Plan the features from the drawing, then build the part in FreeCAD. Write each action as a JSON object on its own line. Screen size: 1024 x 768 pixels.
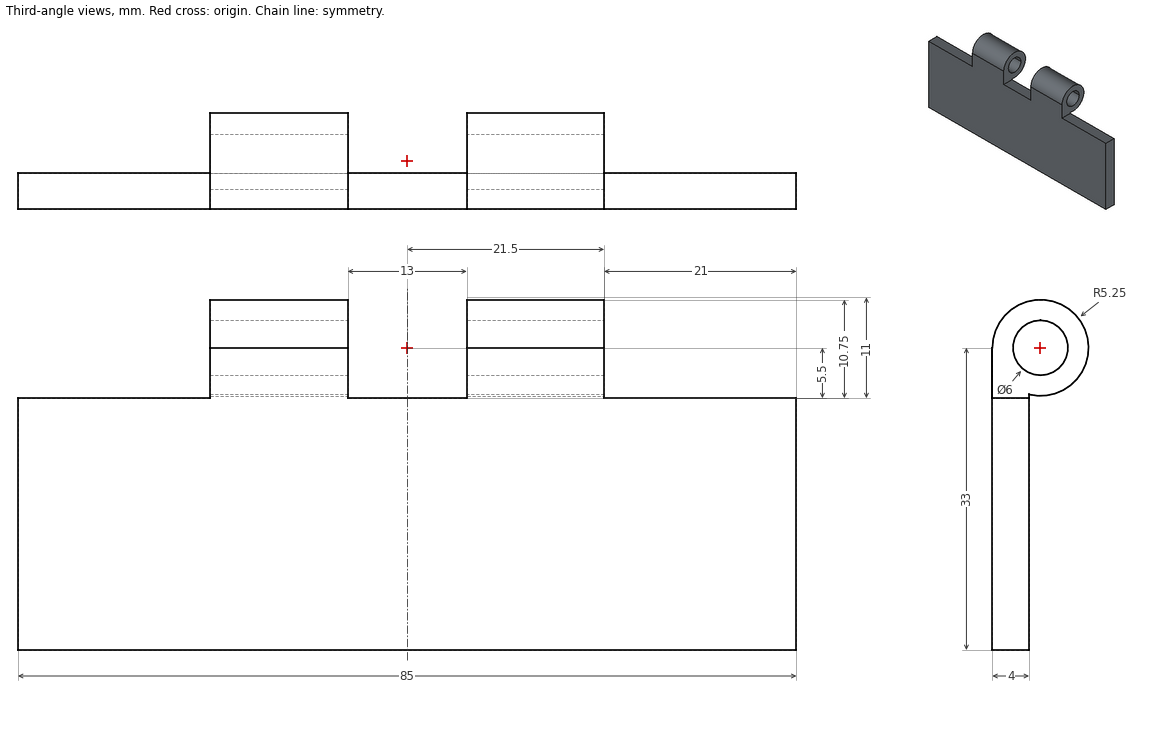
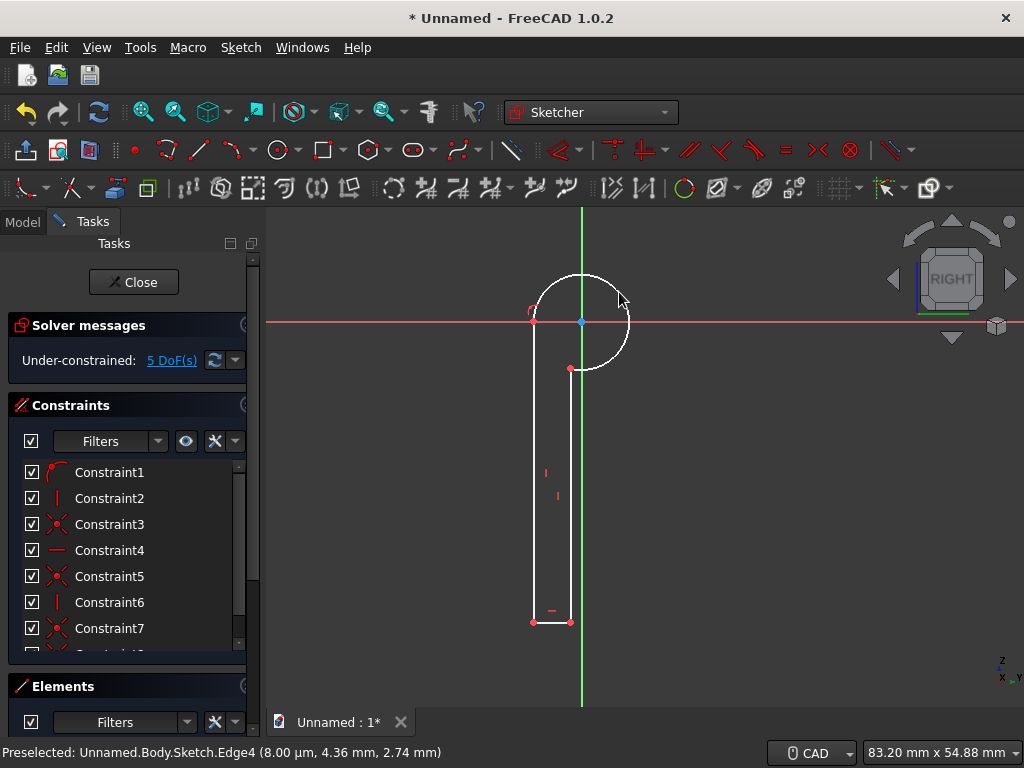
{"action": "left_click", "coordinate": [534, 412]}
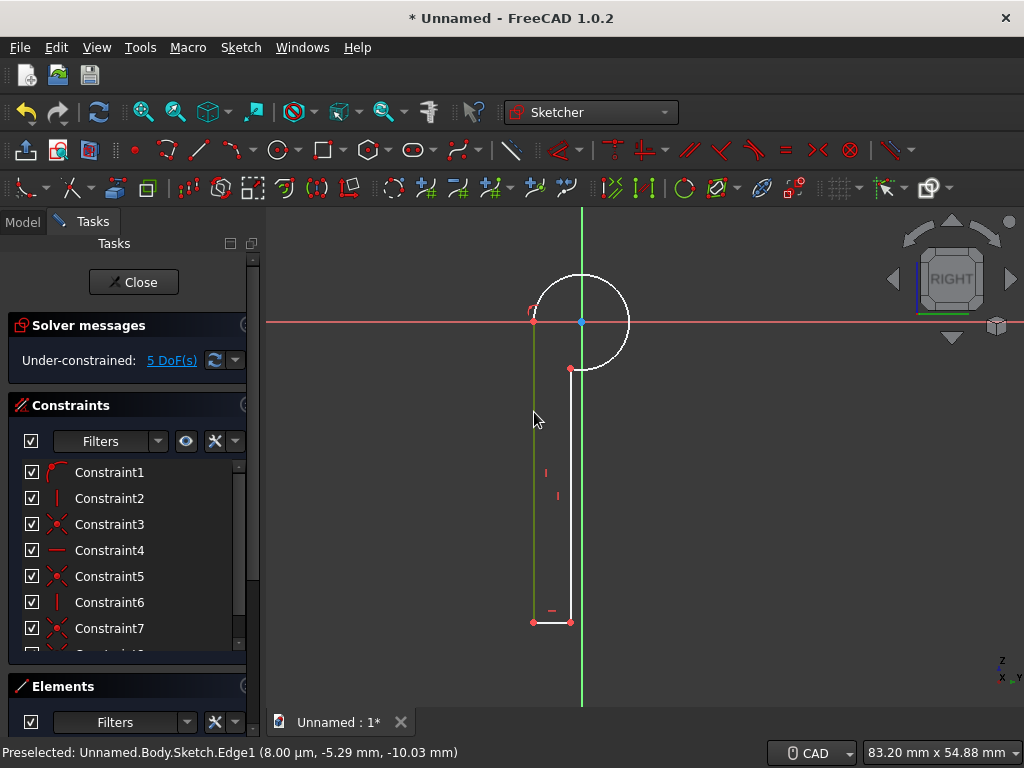
{"action": "left_click", "coordinate": [627, 337]}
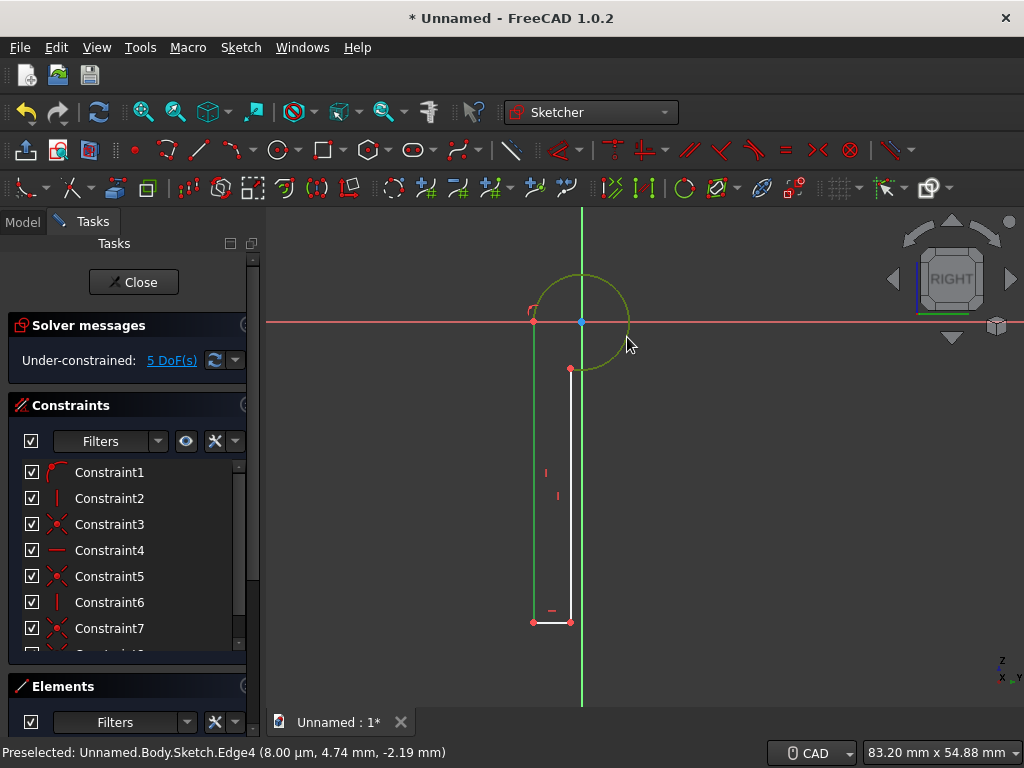
{"action": "left_click", "coordinate": [754, 150]}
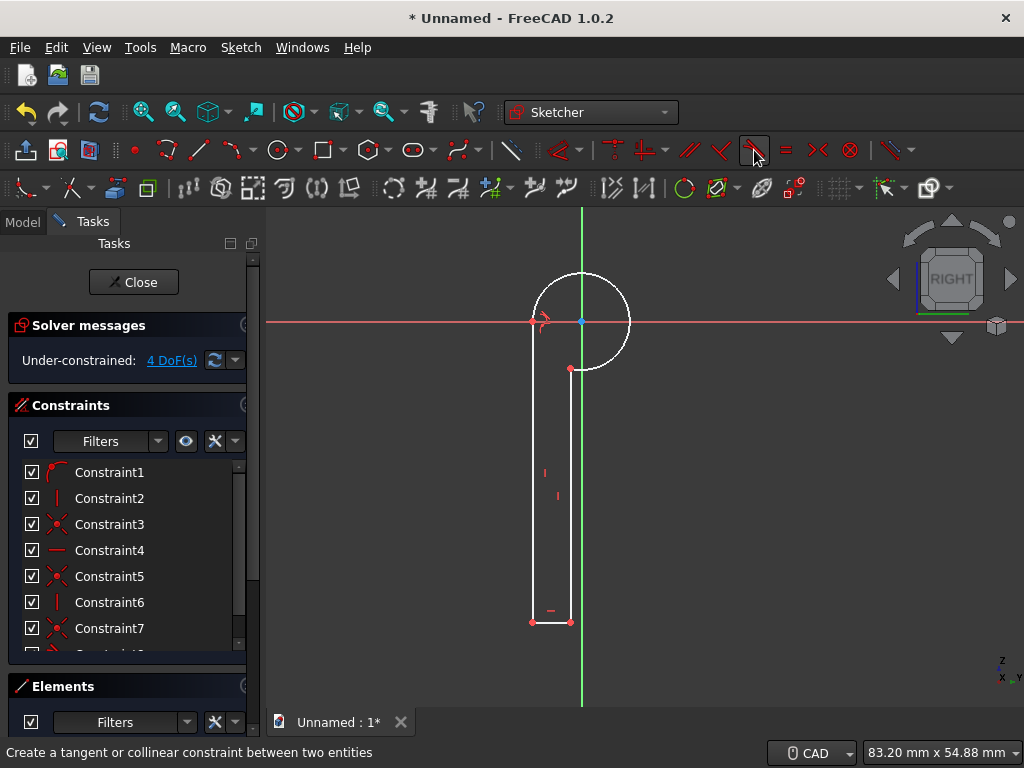
{"action": "left_click", "coordinate": [581, 322]}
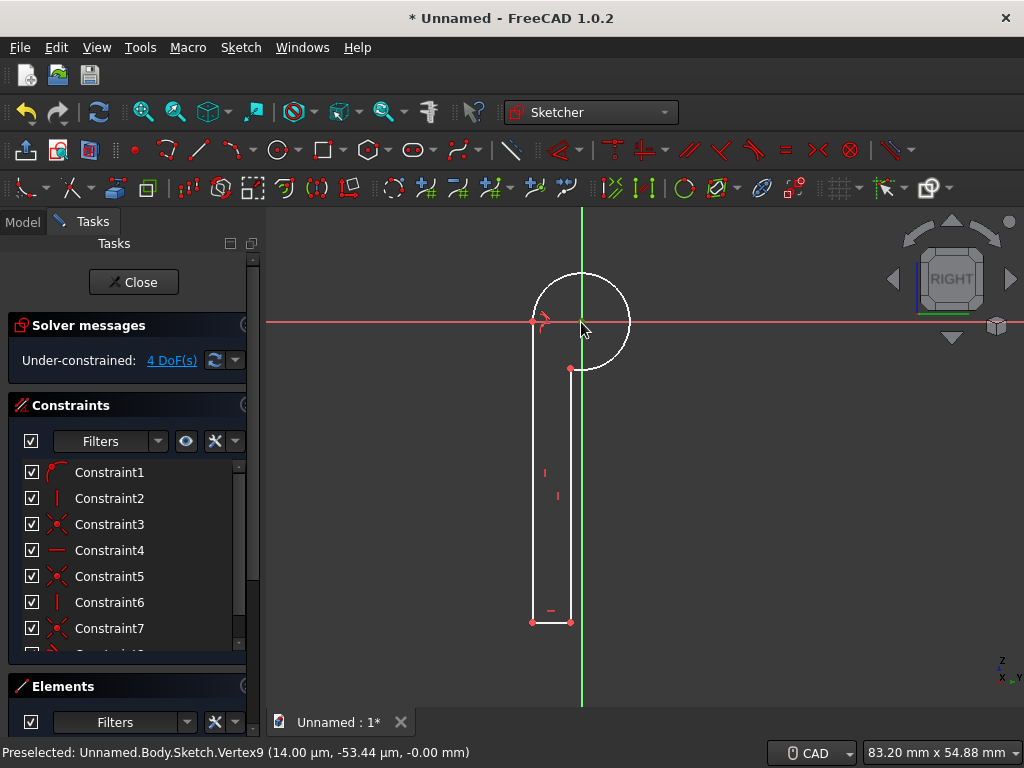
{"action": "left_click", "coordinate": [582, 647]}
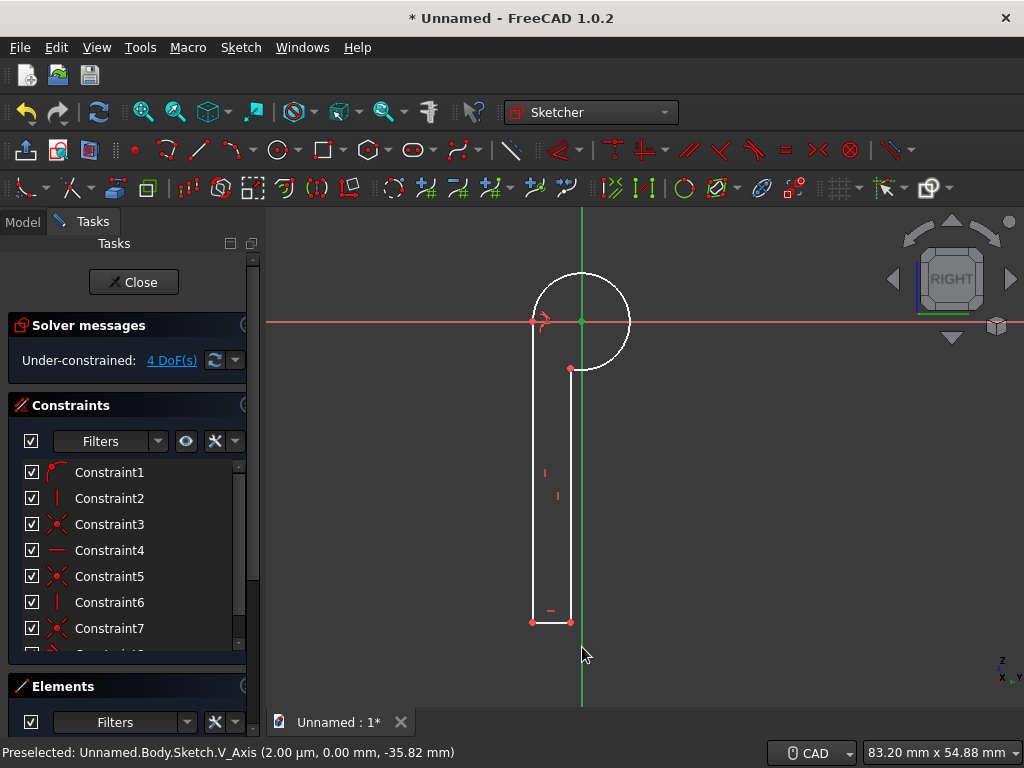
{"action": "left_click", "coordinate": [614, 150]}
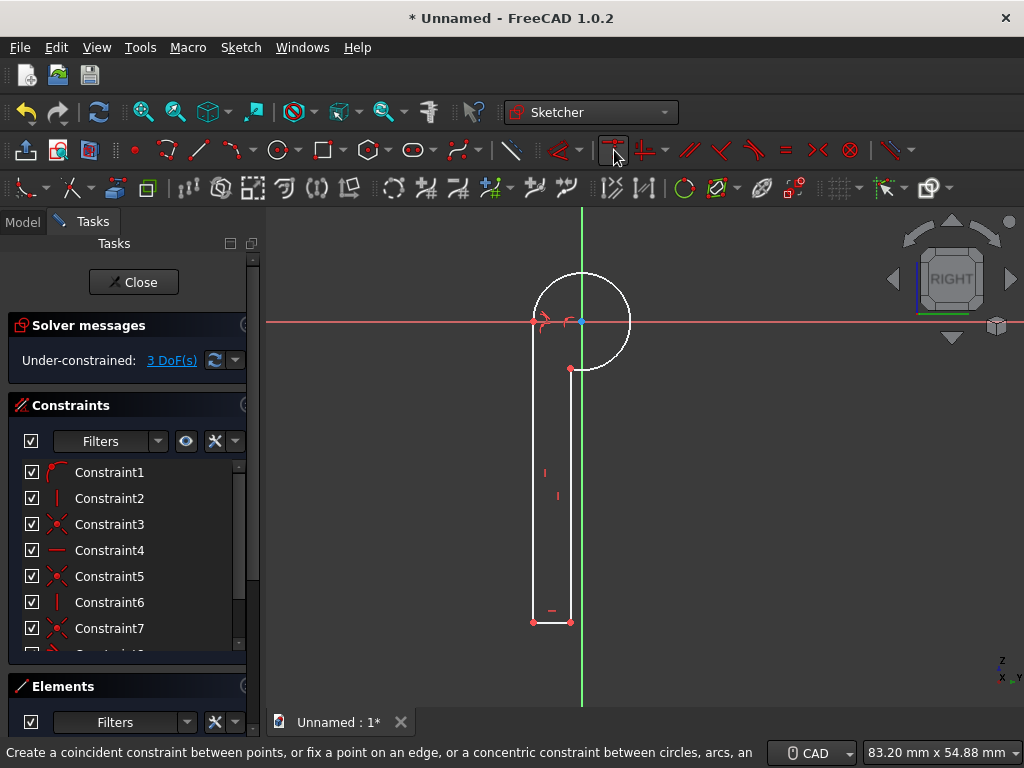
{"action": "left_click", "coordinate": [628, 337]}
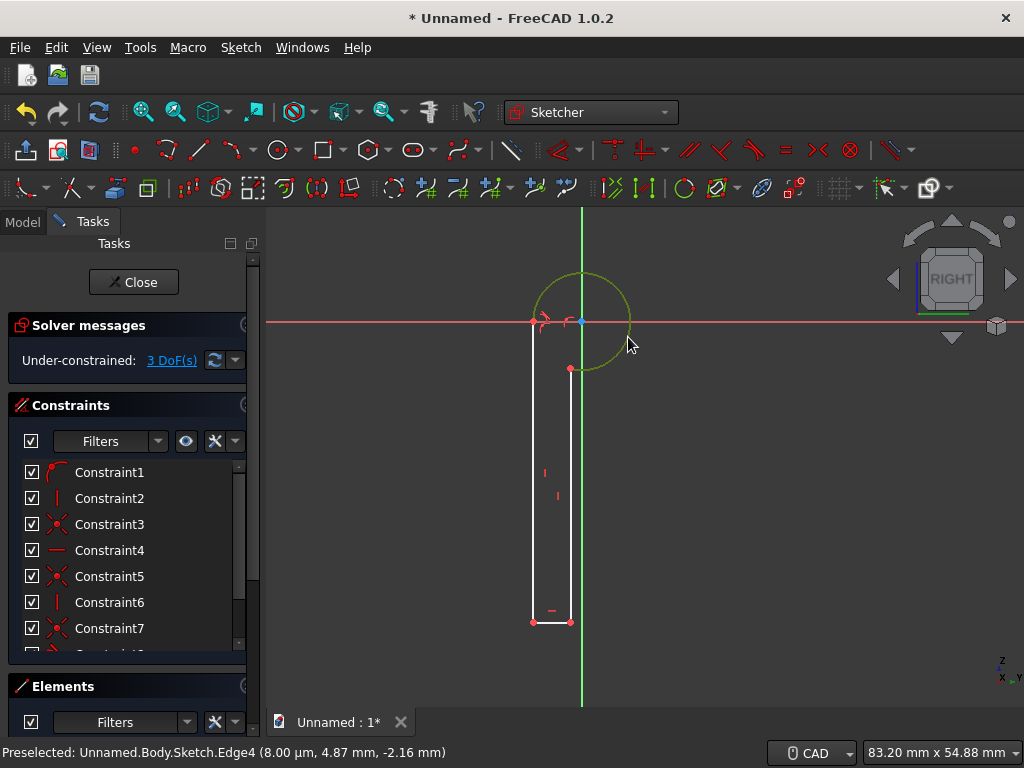
{"action": "key", "text": "k r"}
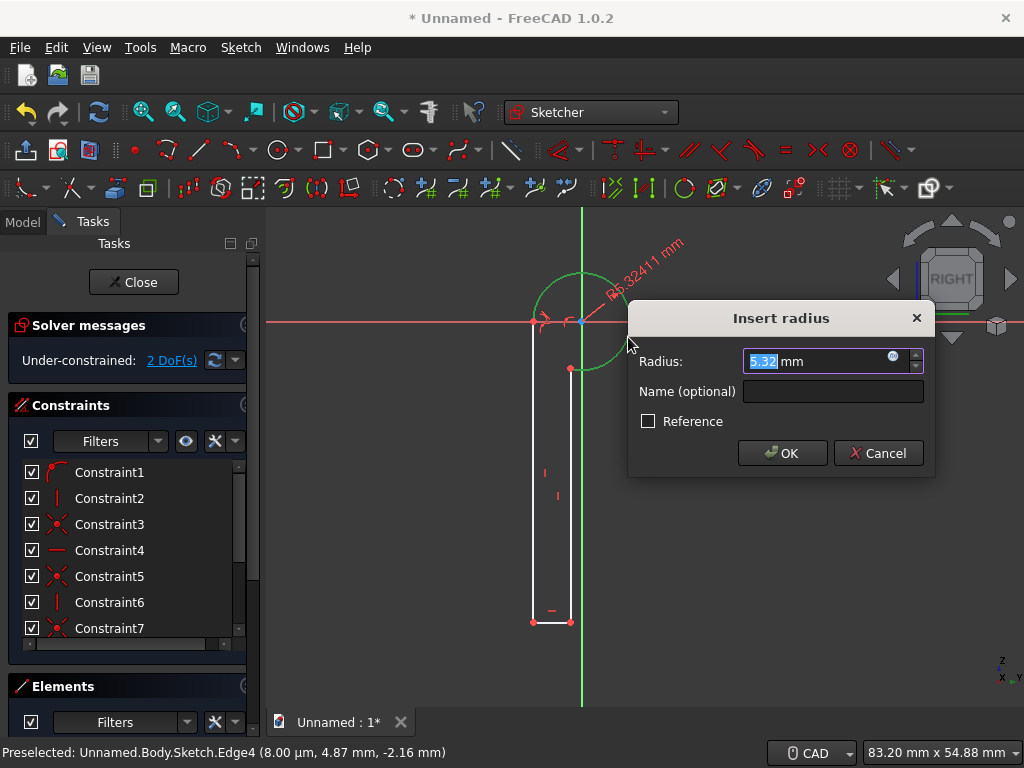
{"action": "type", "text": "5.25"}
{"action": "key", "text": "Return"}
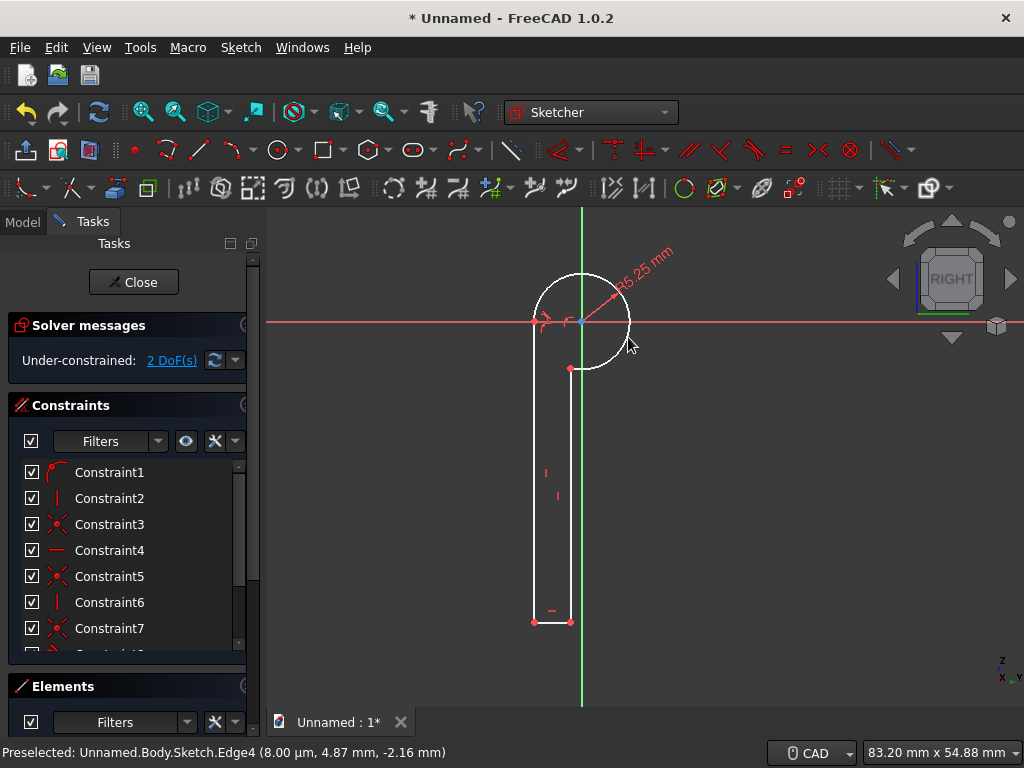
{"action": "scroll", "coordinate": [545, 623], "scroll_direction": "up", "scroll_amount": 2}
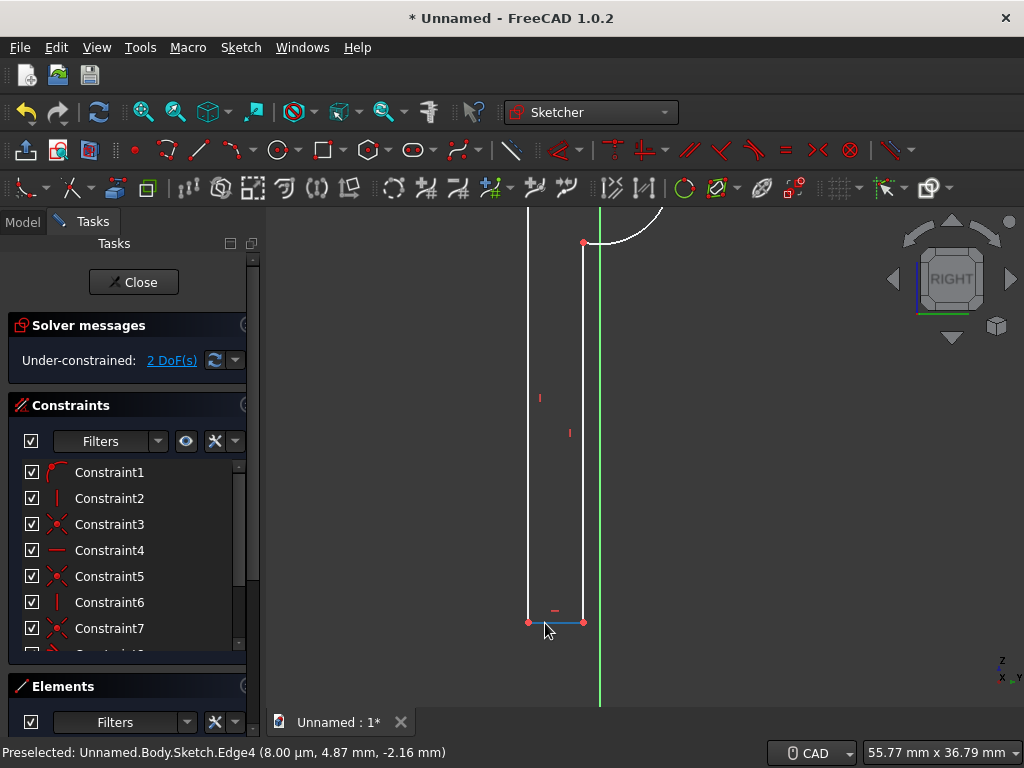
{"action": "left_click", "coordinate": [545, 623]}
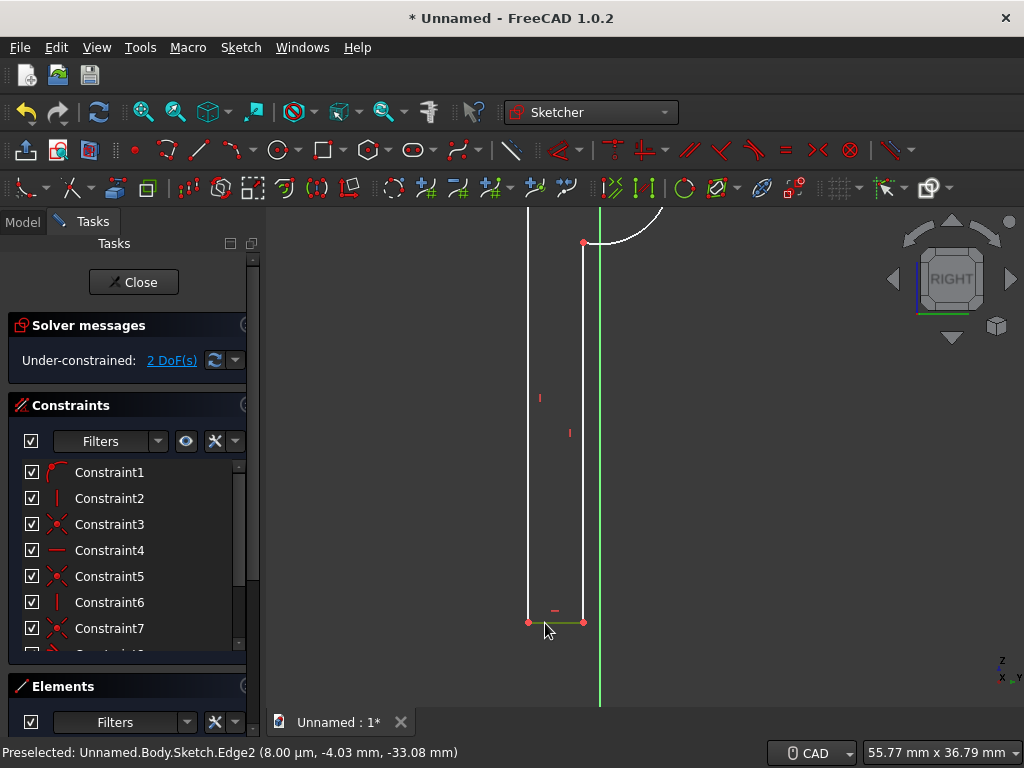
{"action": "left_click", "coordinate": [582, 150]}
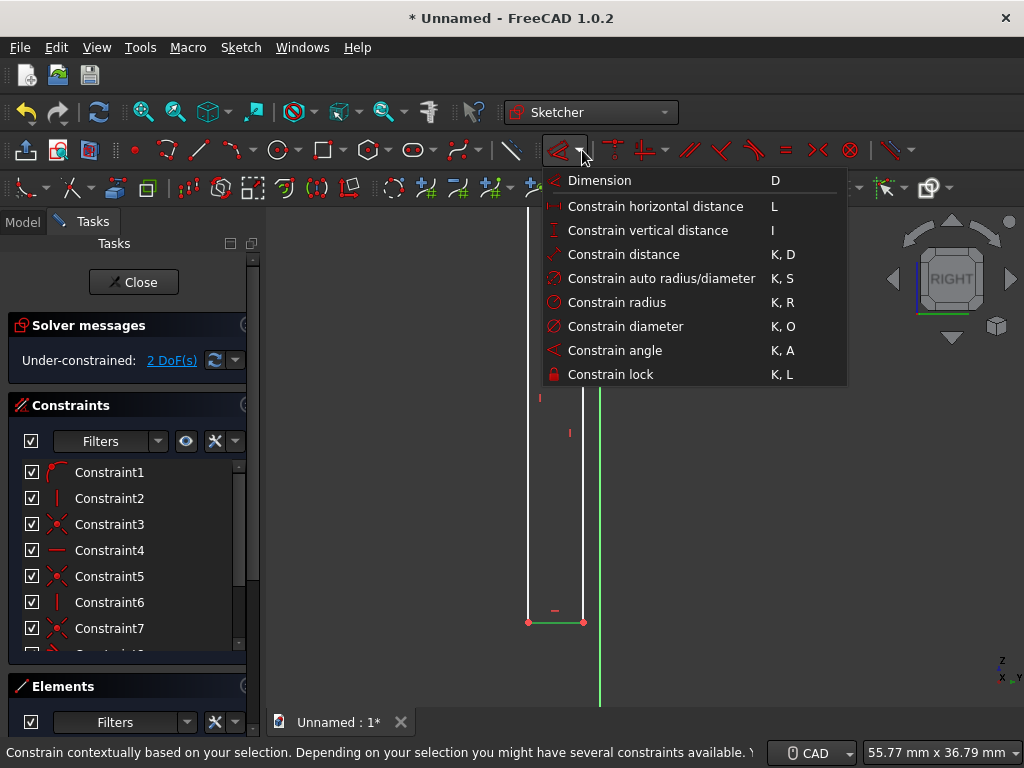
{"action": "left_click", "coordinate": [695, 206]}